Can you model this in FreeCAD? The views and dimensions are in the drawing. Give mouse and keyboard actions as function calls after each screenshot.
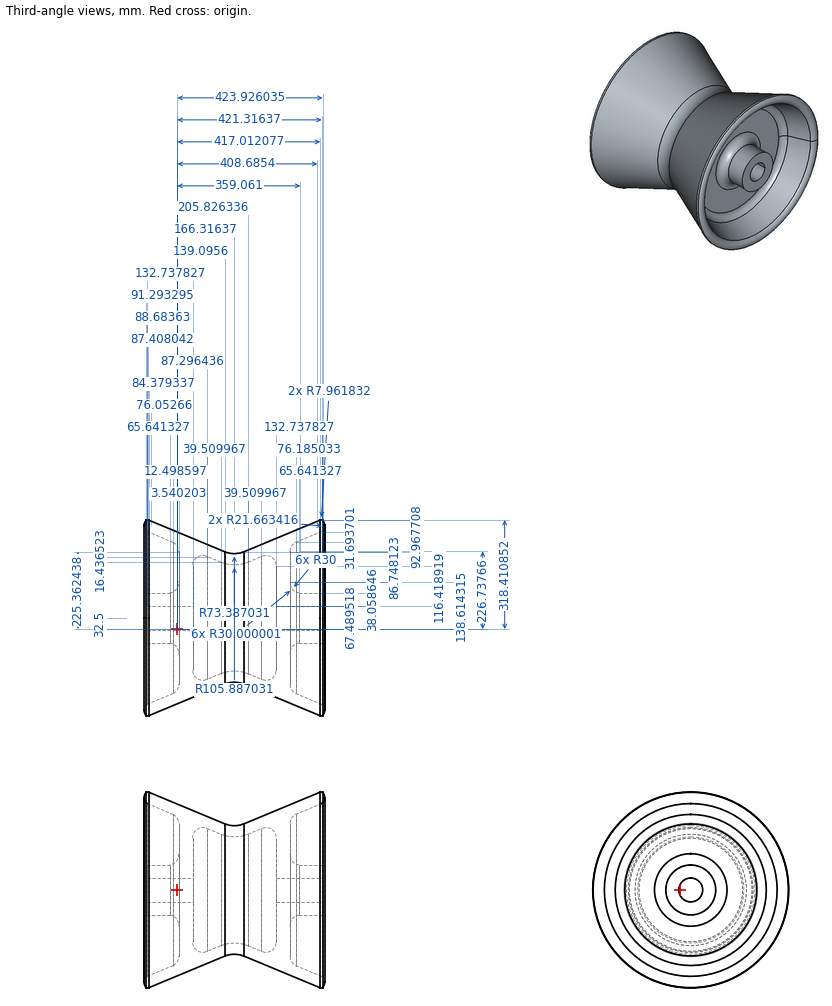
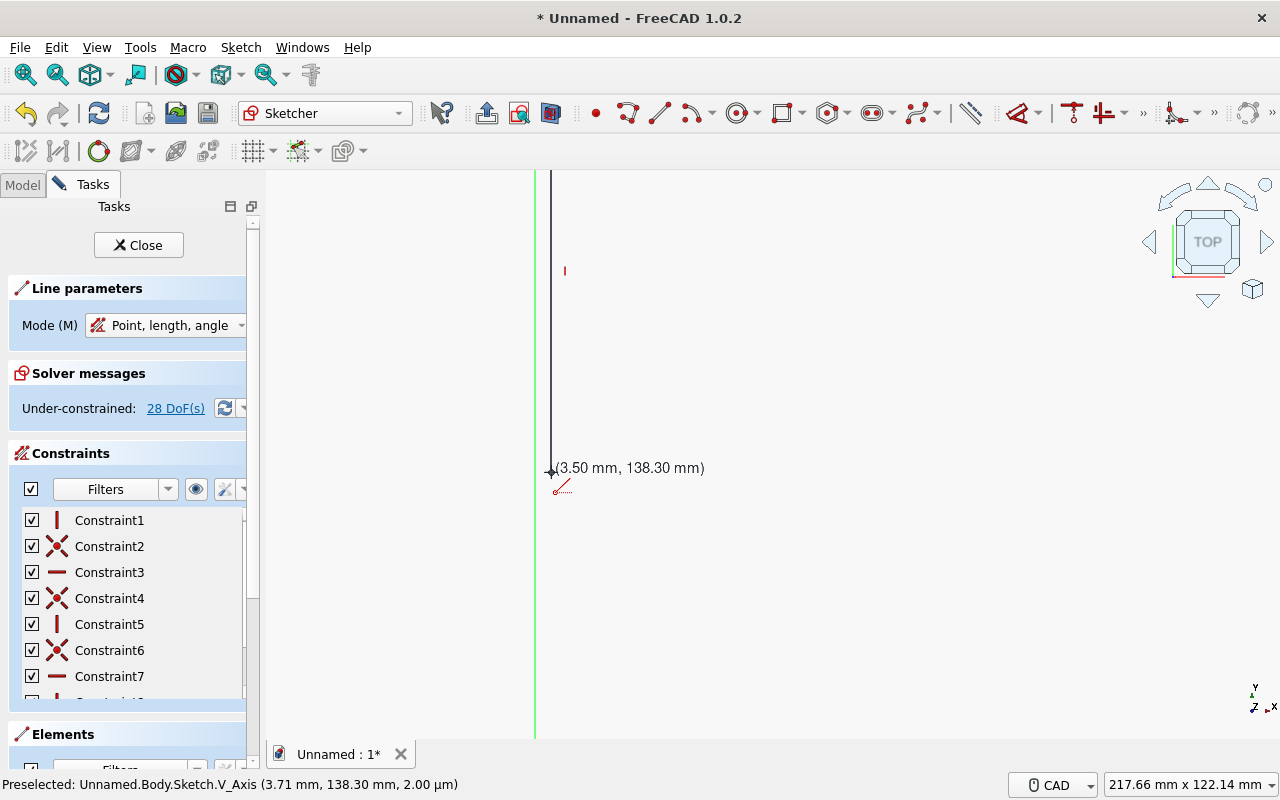
key(g)
key(m)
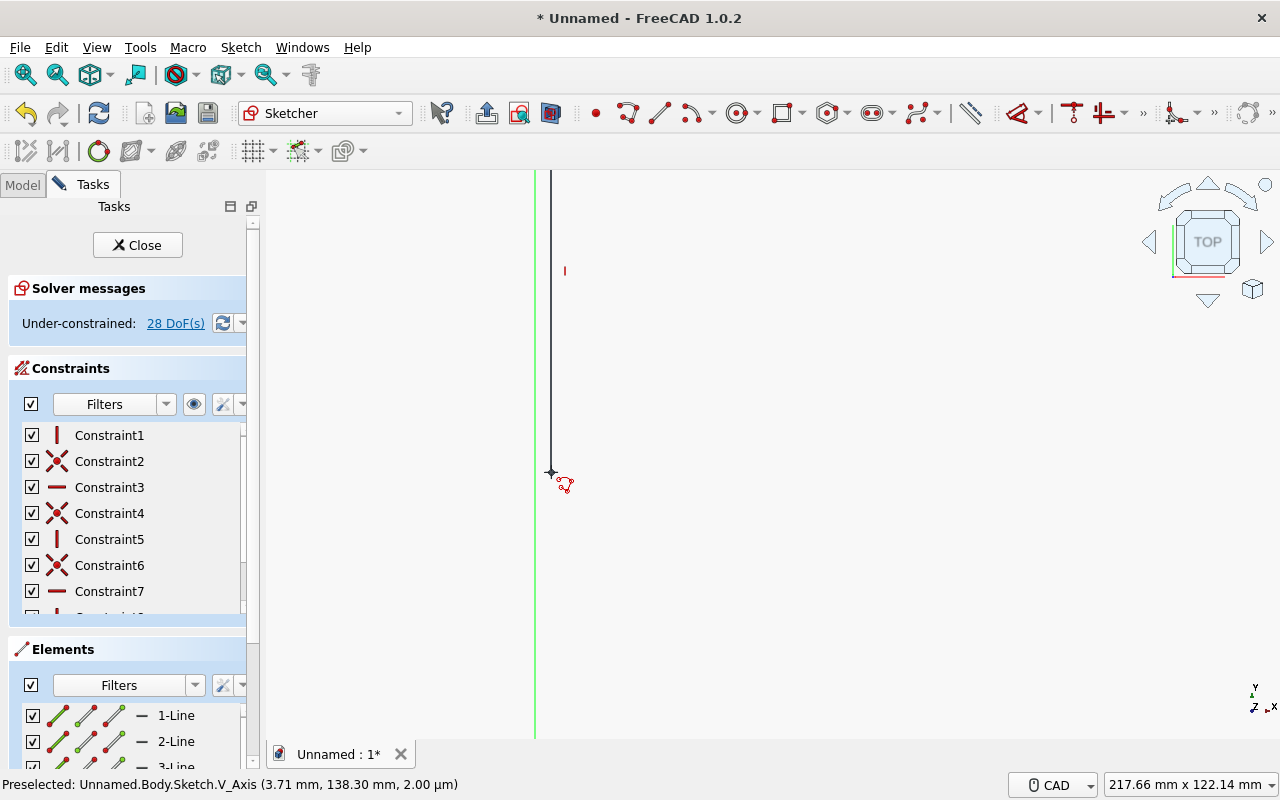
scroll(551, 475, down, 8)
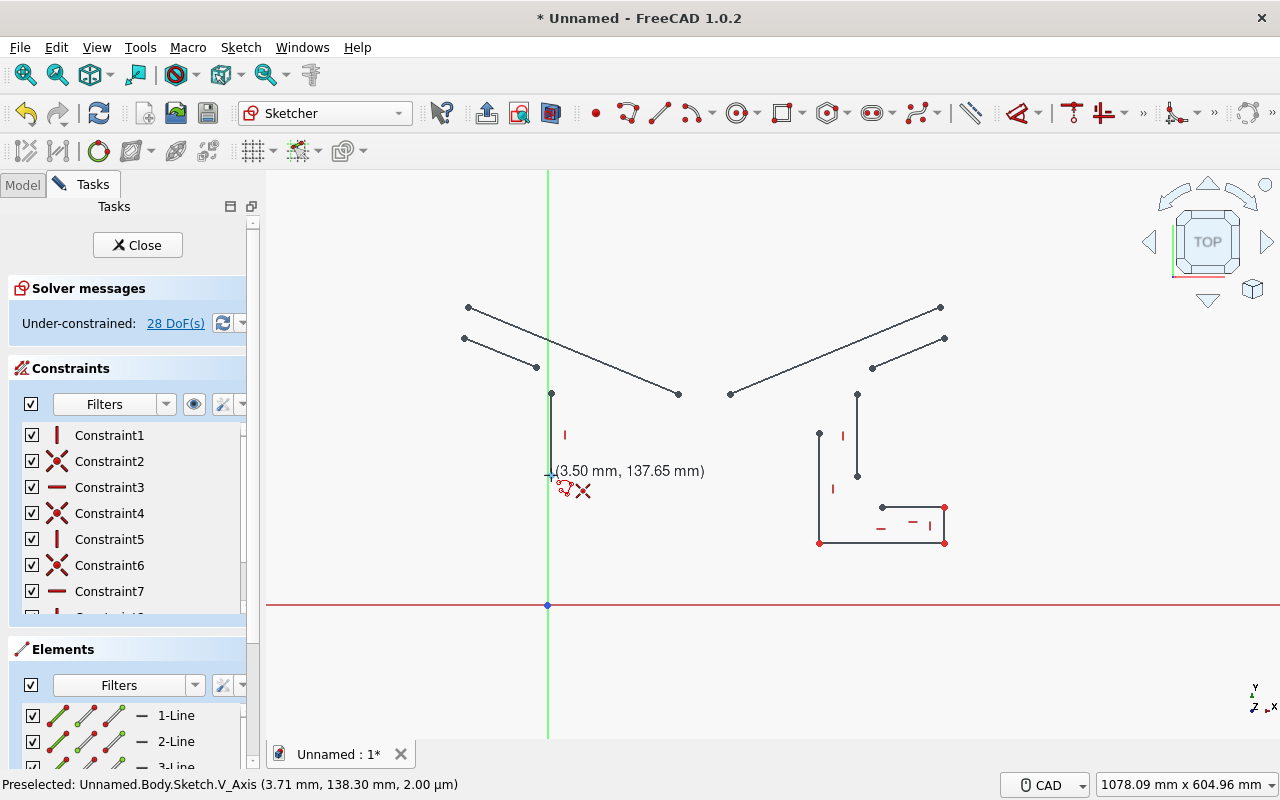
click(526, 506)
click(465, 506)
click(465, 542)
click(589, 542)
click(589, 432)
right_click(589, 432)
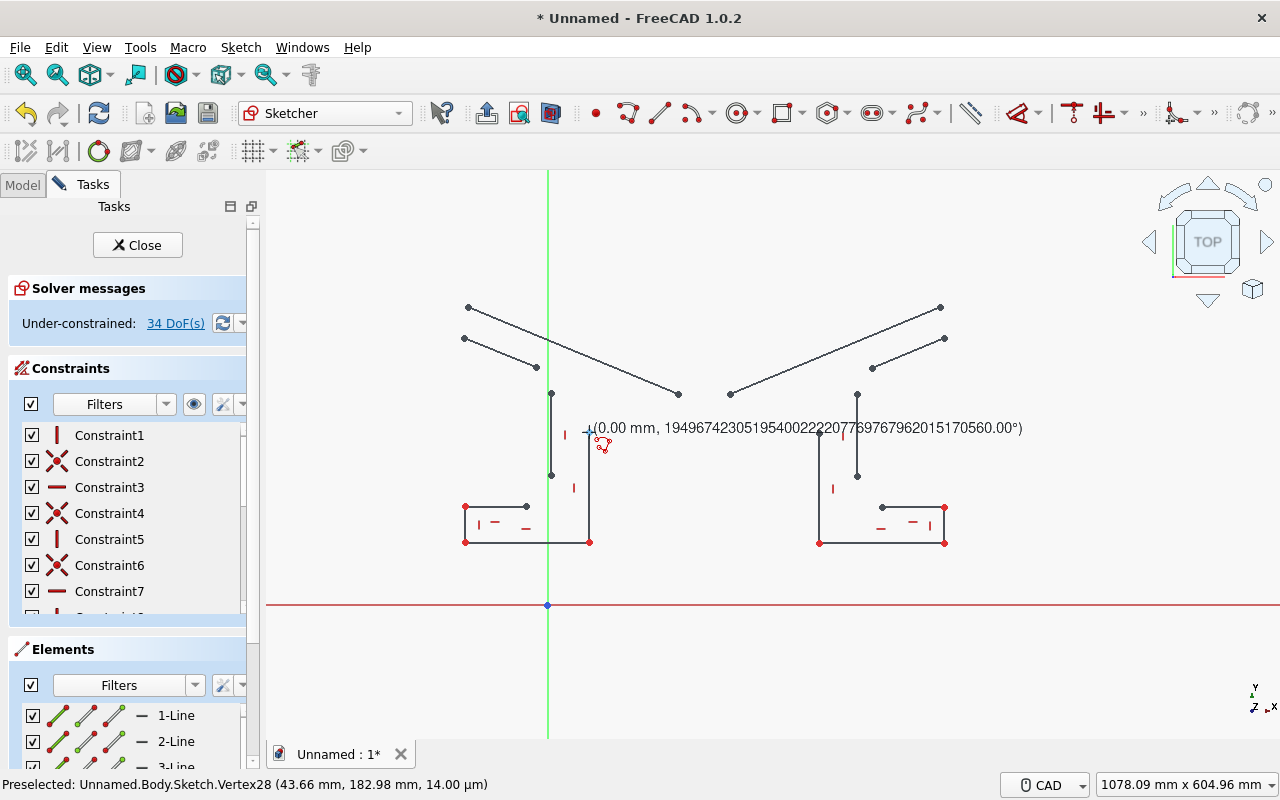
click(660, 114)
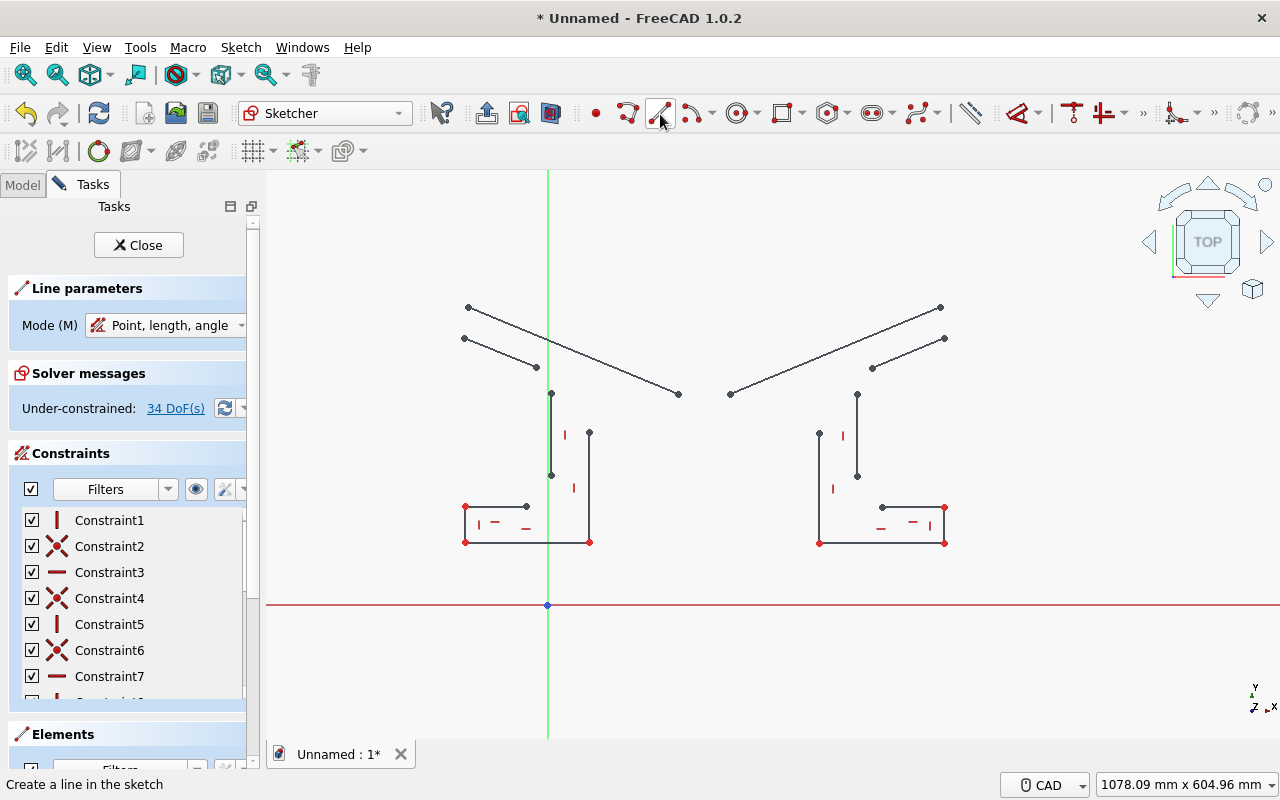
click(630, 406)
click(667, 421)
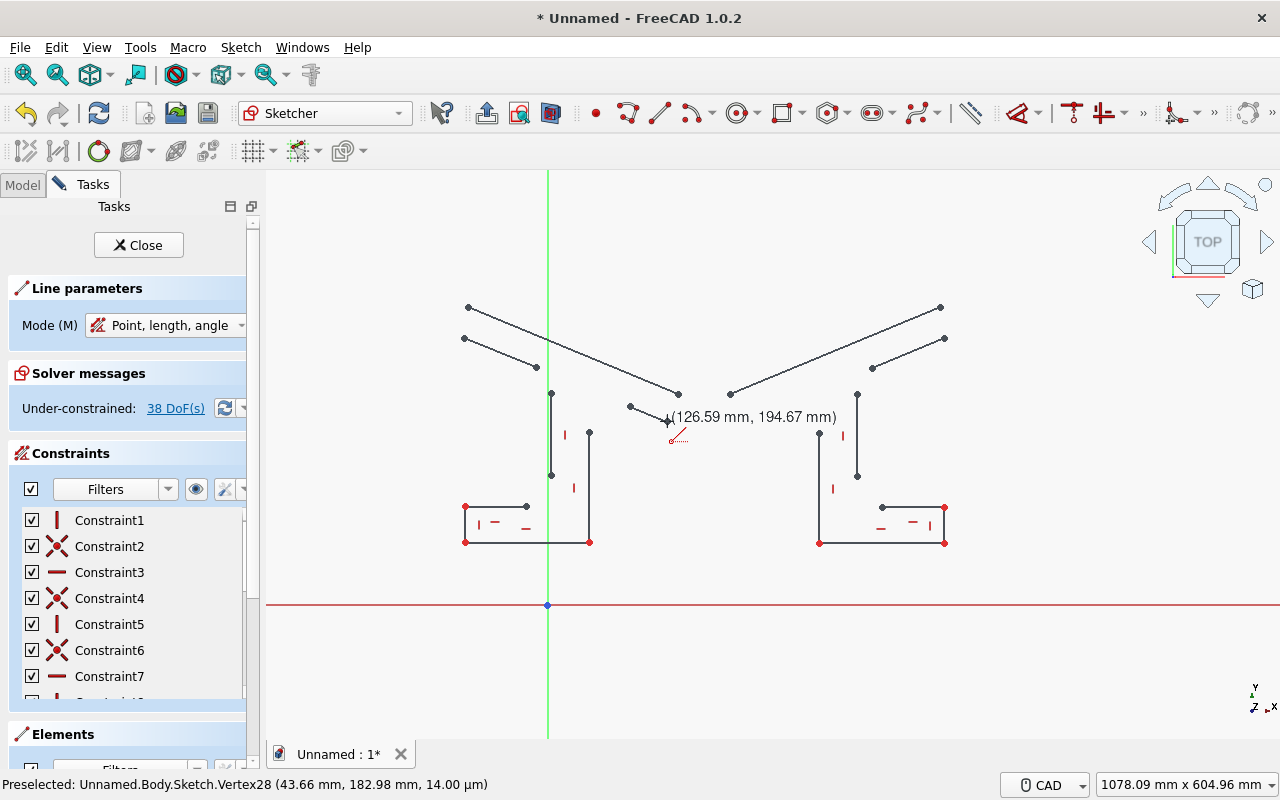
click(742, 421)
click(779, 406)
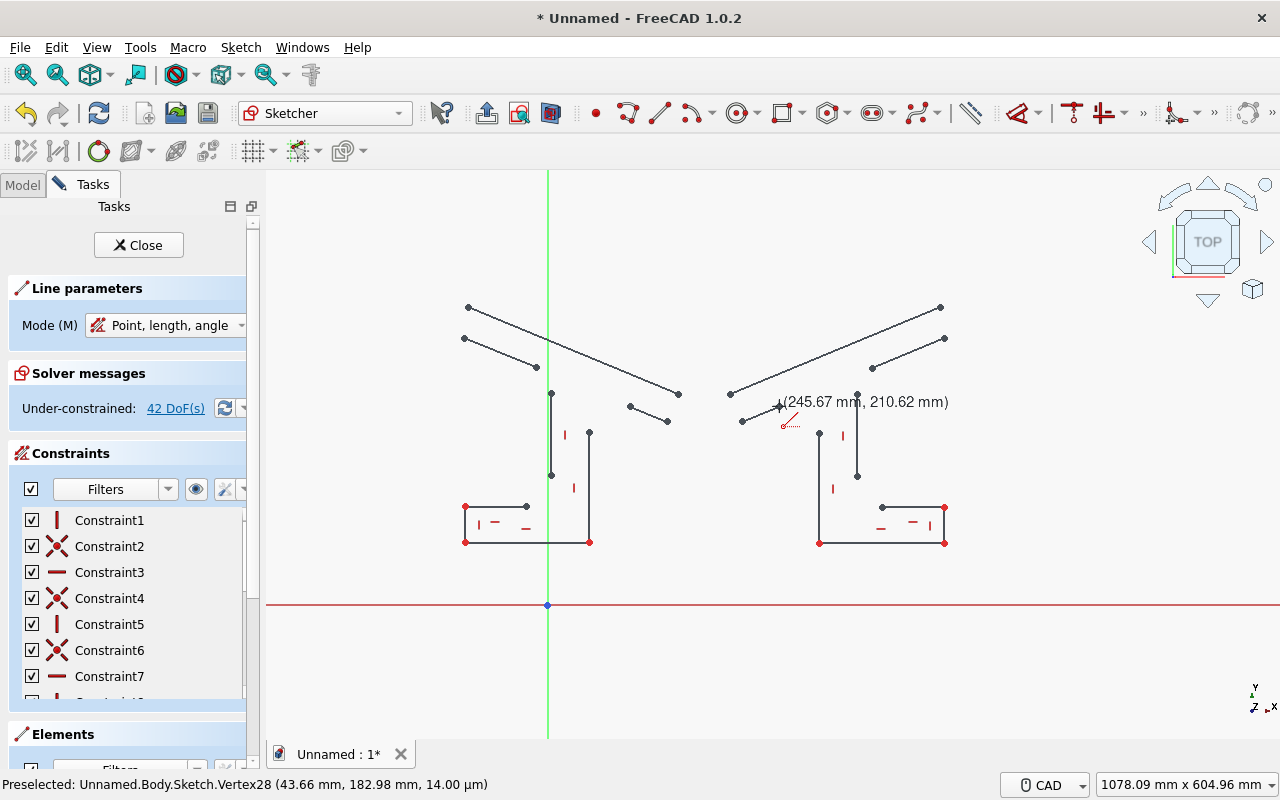
click(714, 114)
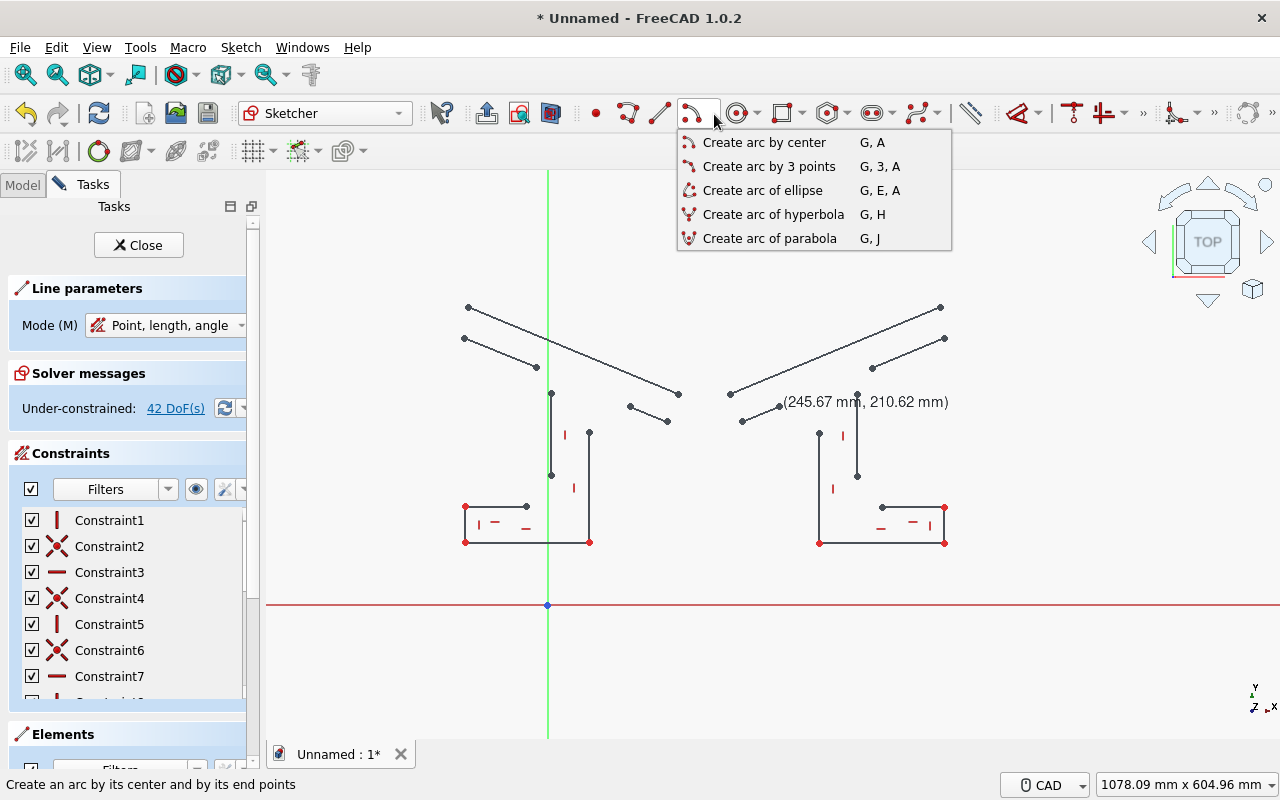
click(814, 166)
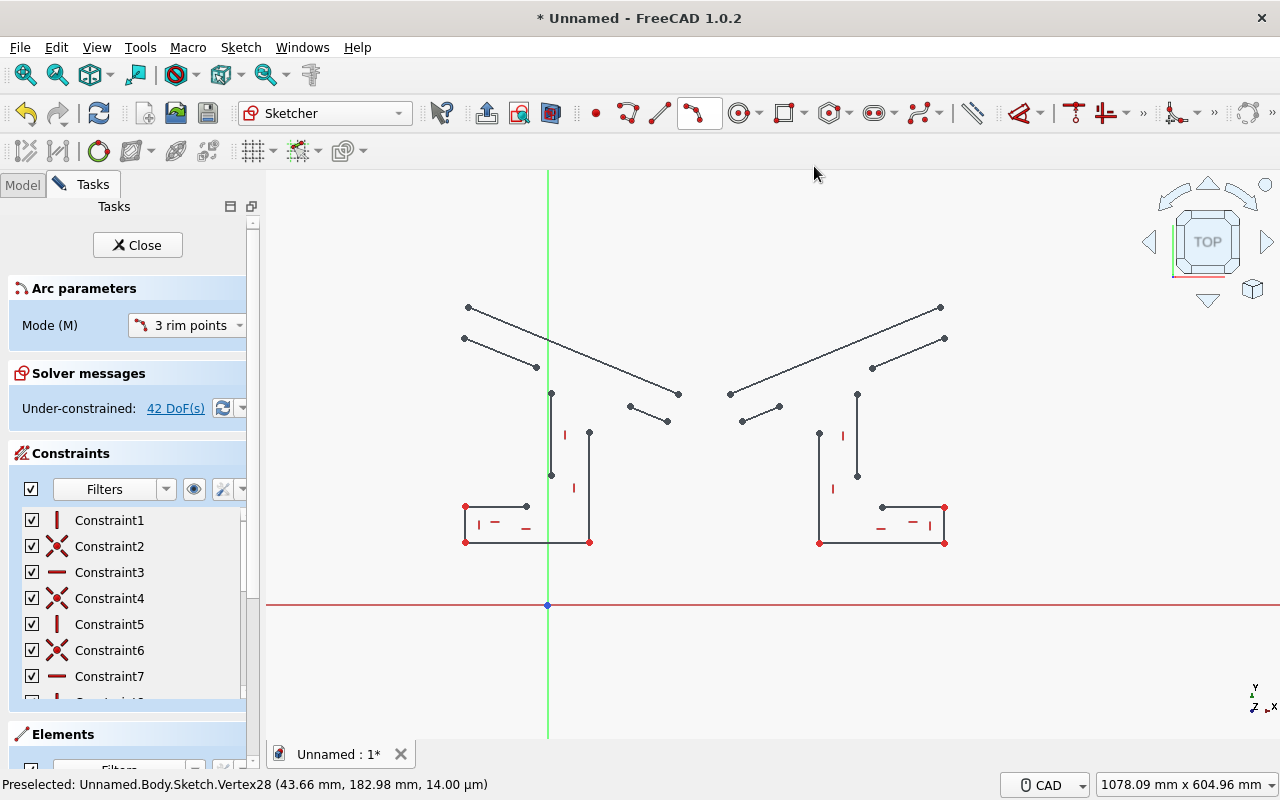
click(882, 507)
click(857, 476)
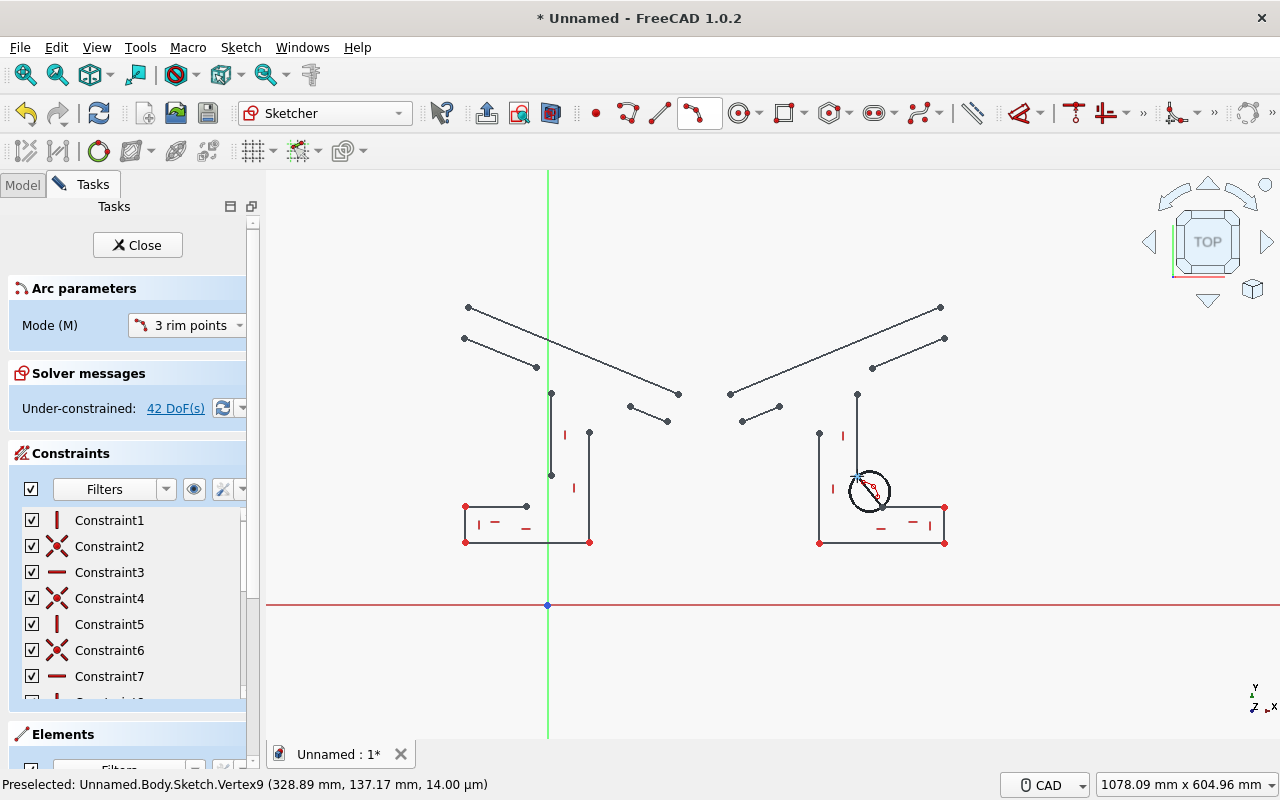
scroll(864, 495, up, 4)